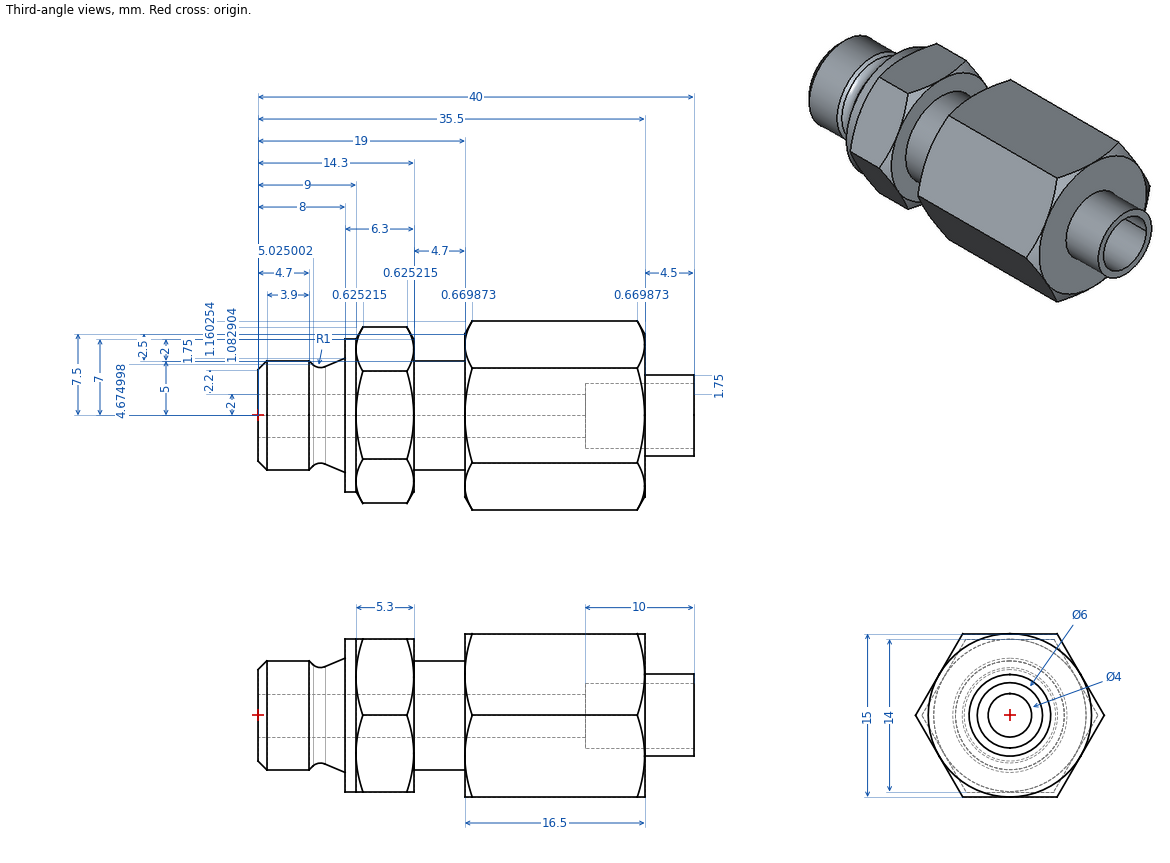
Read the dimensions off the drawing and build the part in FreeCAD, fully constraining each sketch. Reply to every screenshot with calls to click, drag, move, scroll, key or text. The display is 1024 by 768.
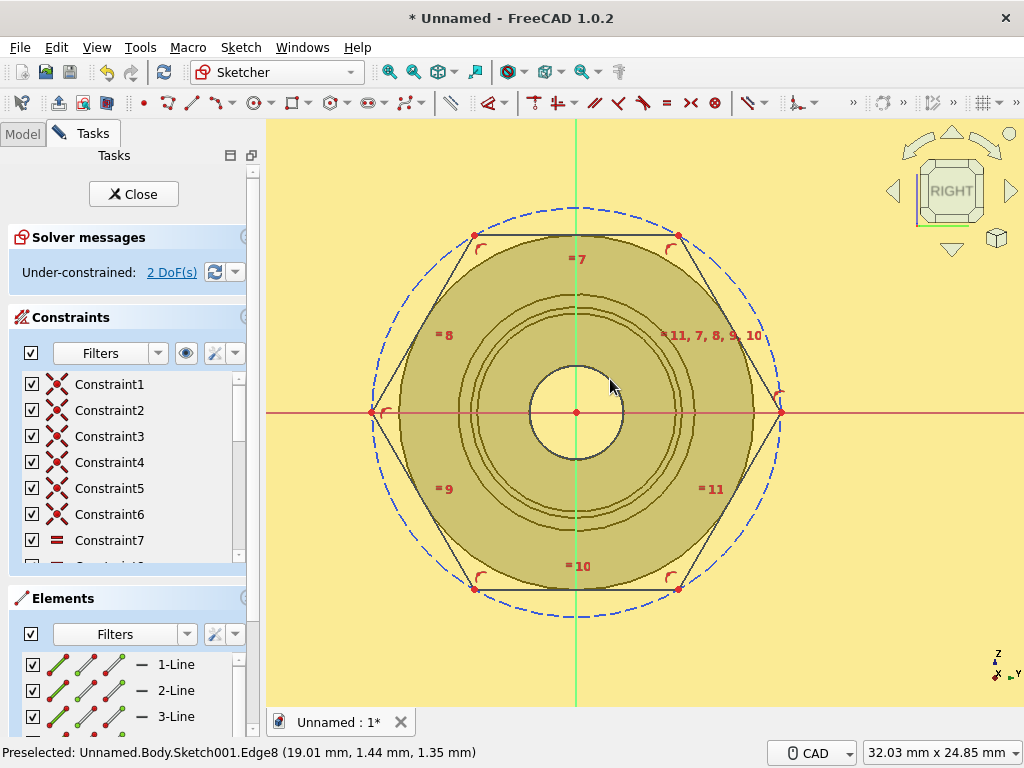
key(d)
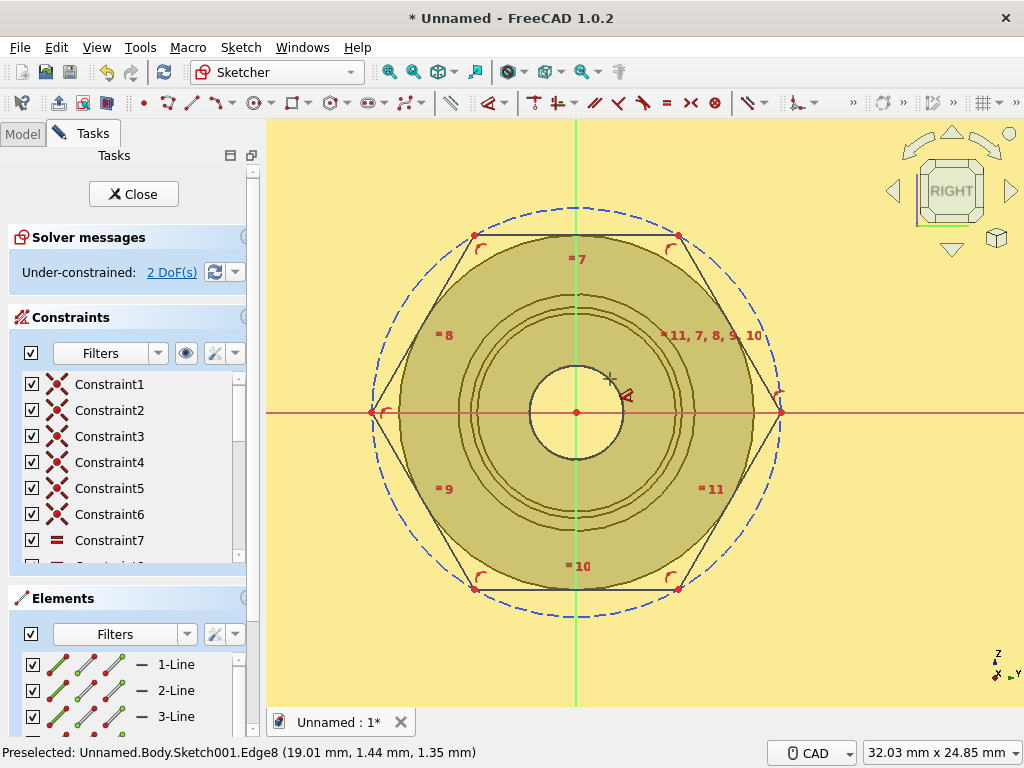
click(609, 379)
click(631, 356)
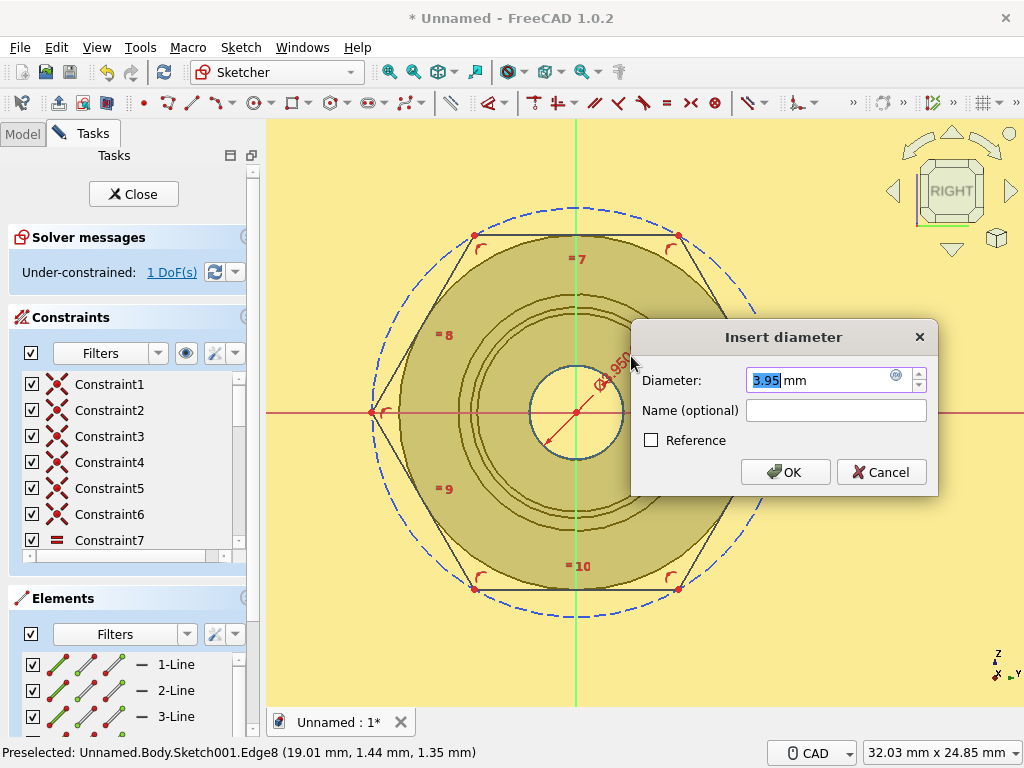
text(4)
key(Return)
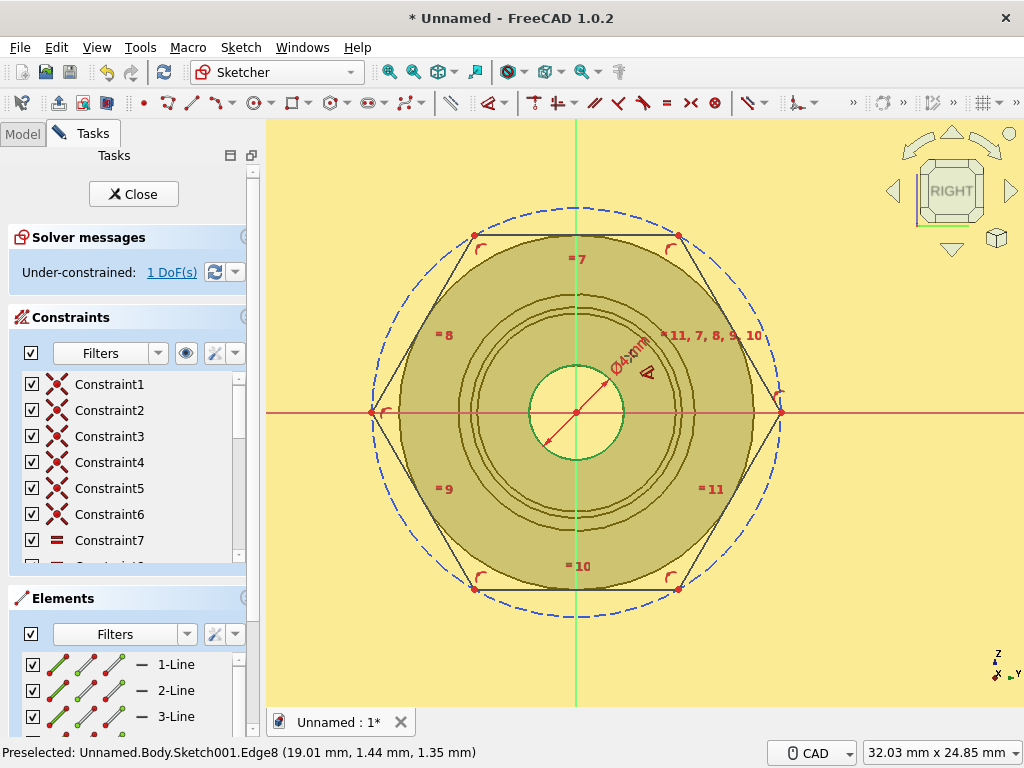
click(474, 590)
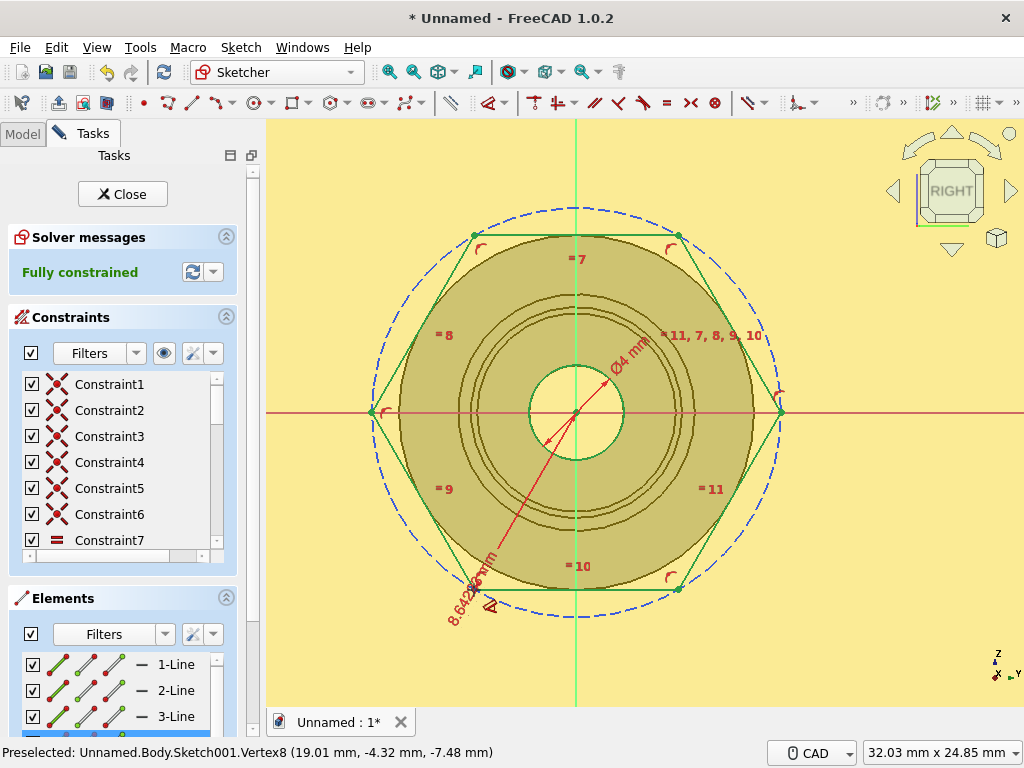
click(679, 235)
click(713, 331)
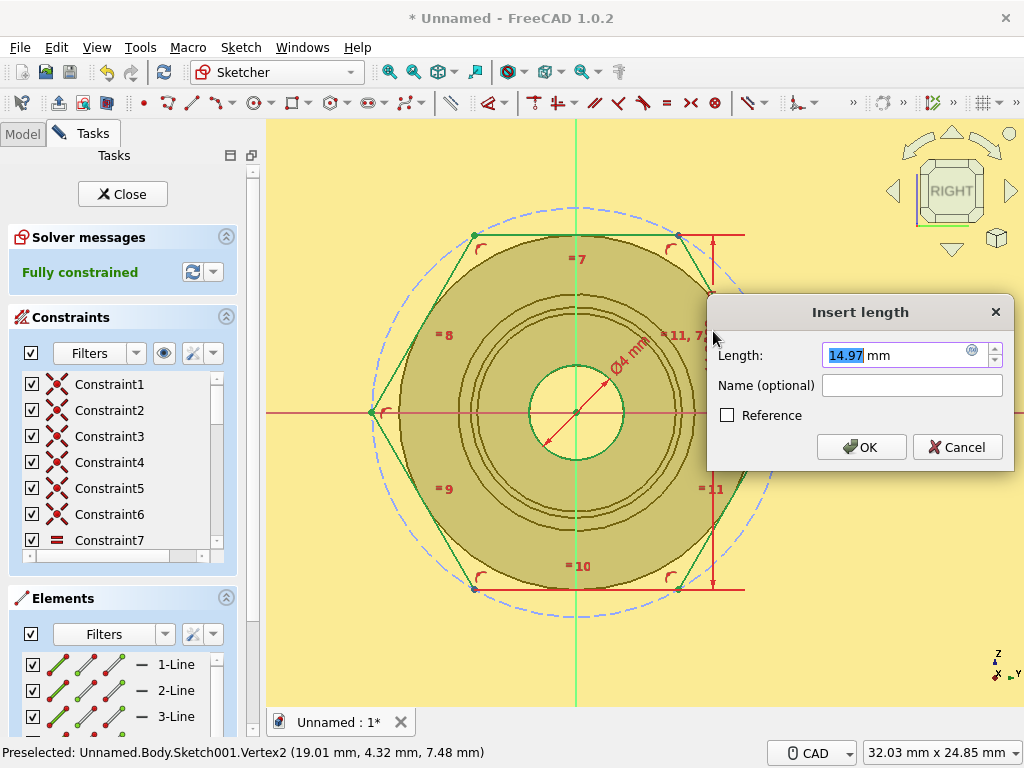
text(15)
key(Return)
key(Escape)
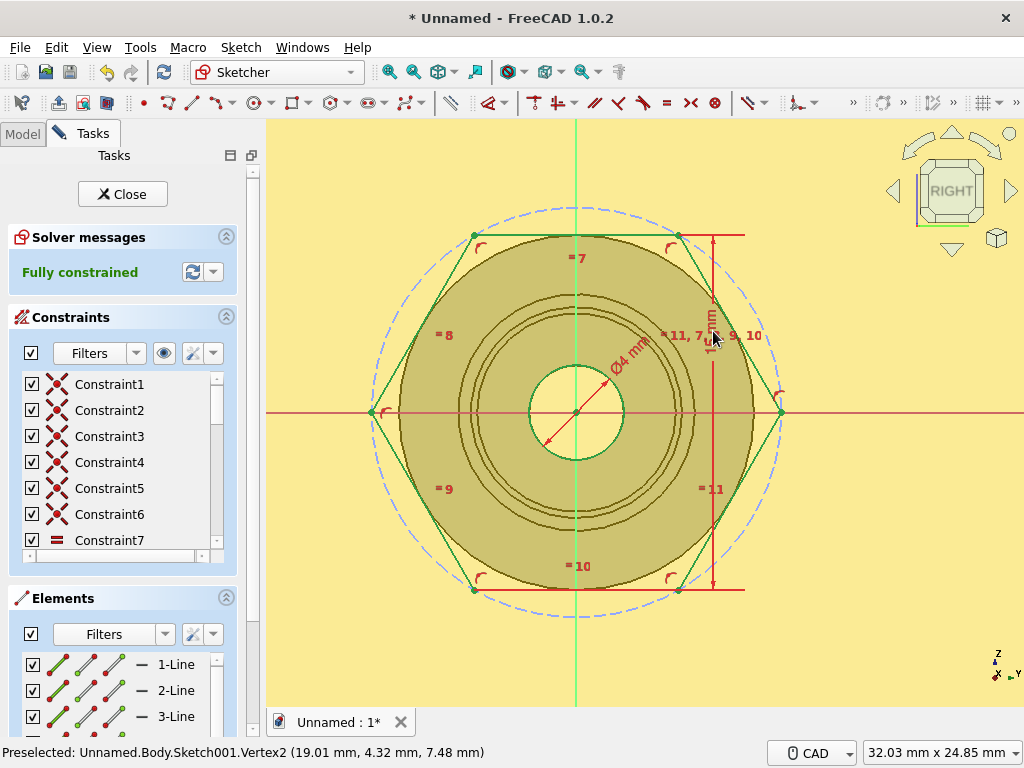
click(123, 194)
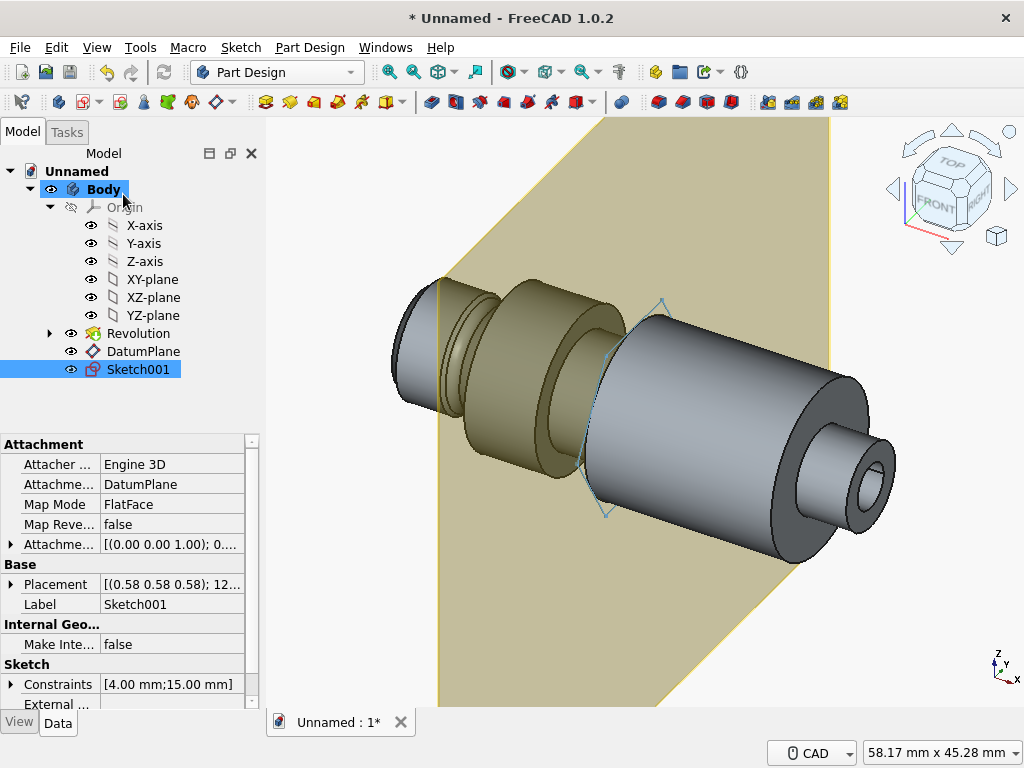
click(266, 102)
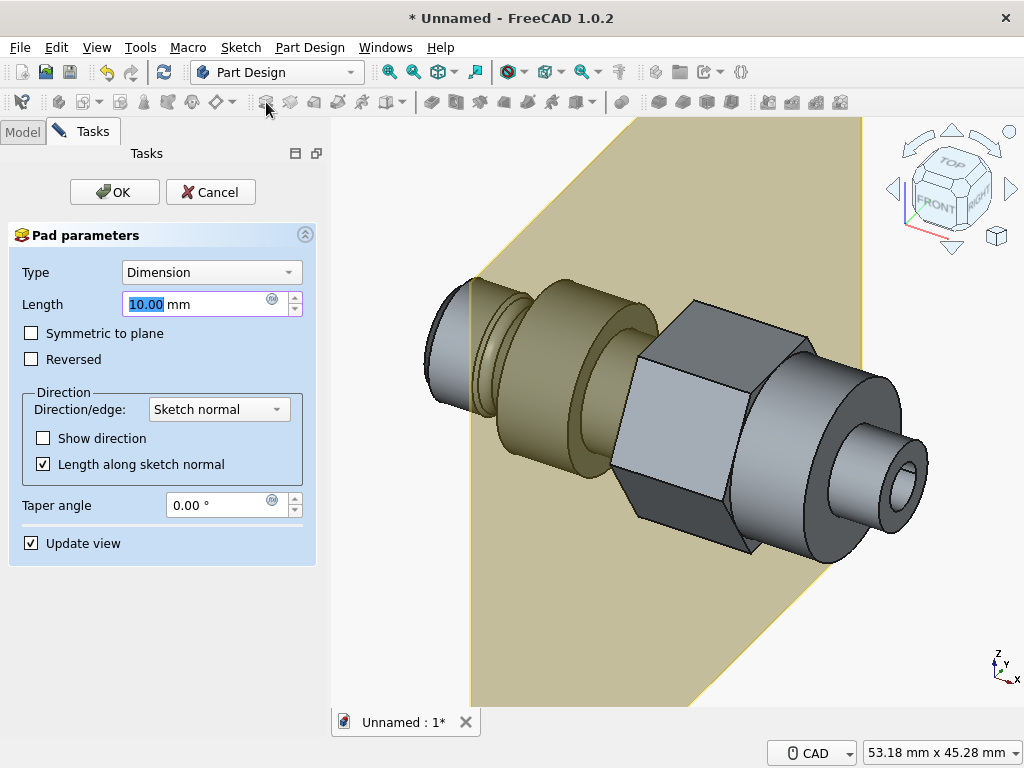
text(16.5)
key(Tab)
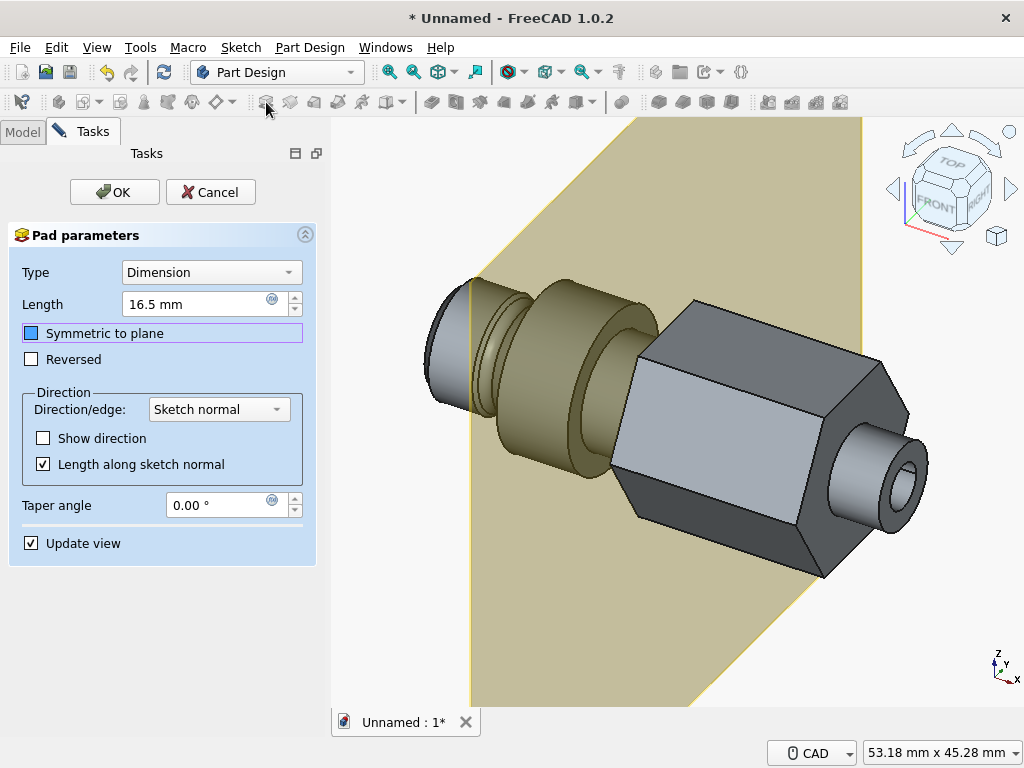
click(115, 192)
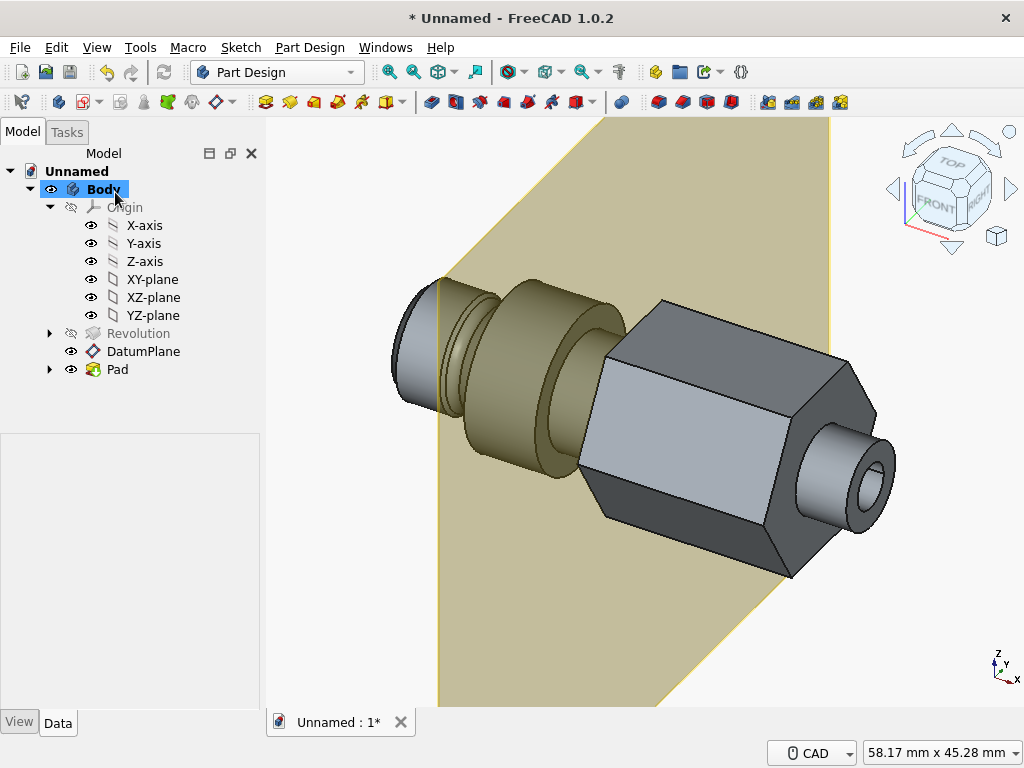
click(116, 351)
key(space)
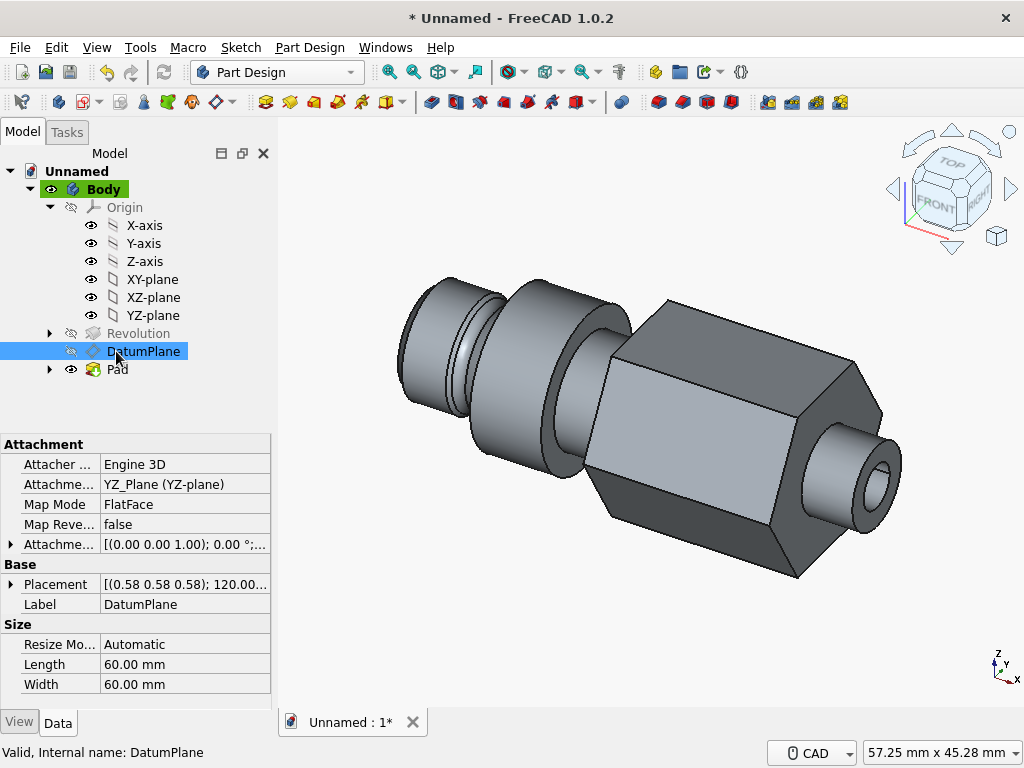
click(136, 315)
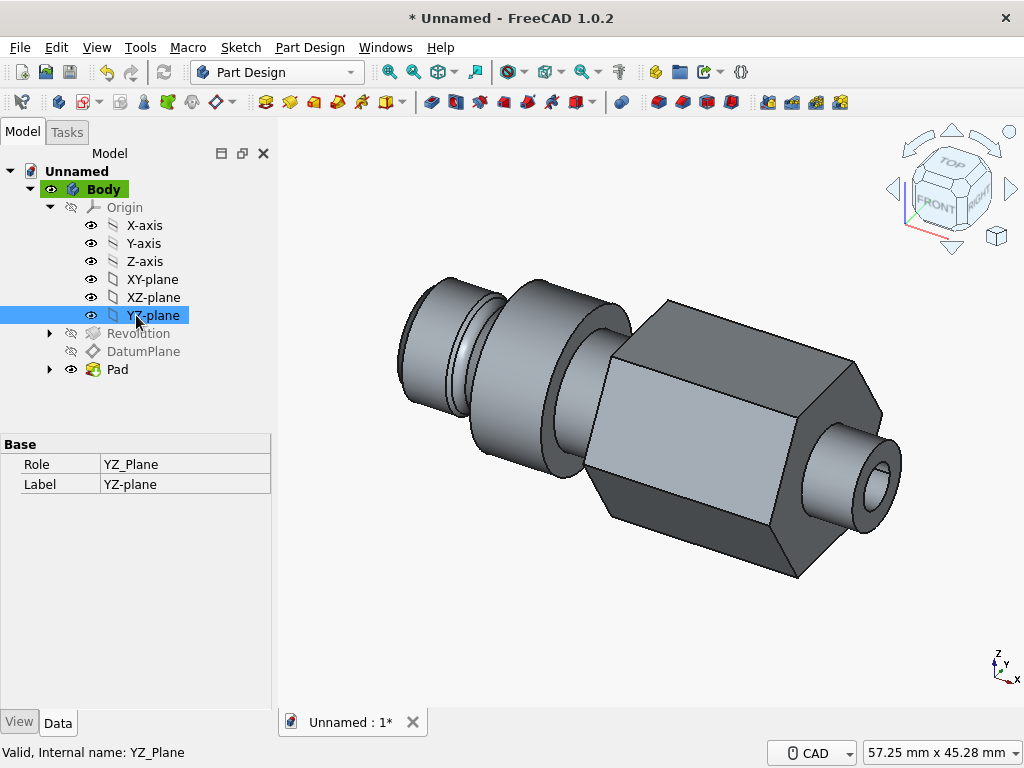
click(216, 102)